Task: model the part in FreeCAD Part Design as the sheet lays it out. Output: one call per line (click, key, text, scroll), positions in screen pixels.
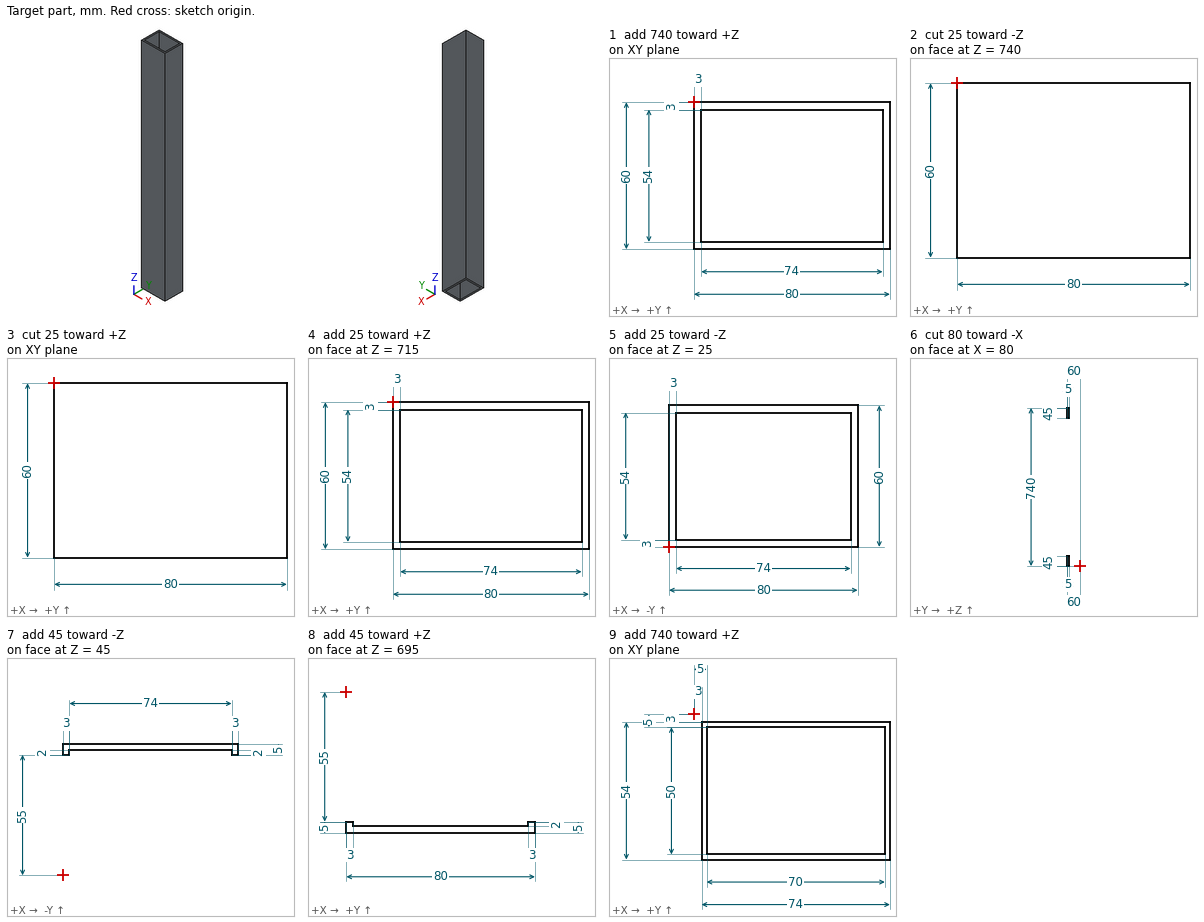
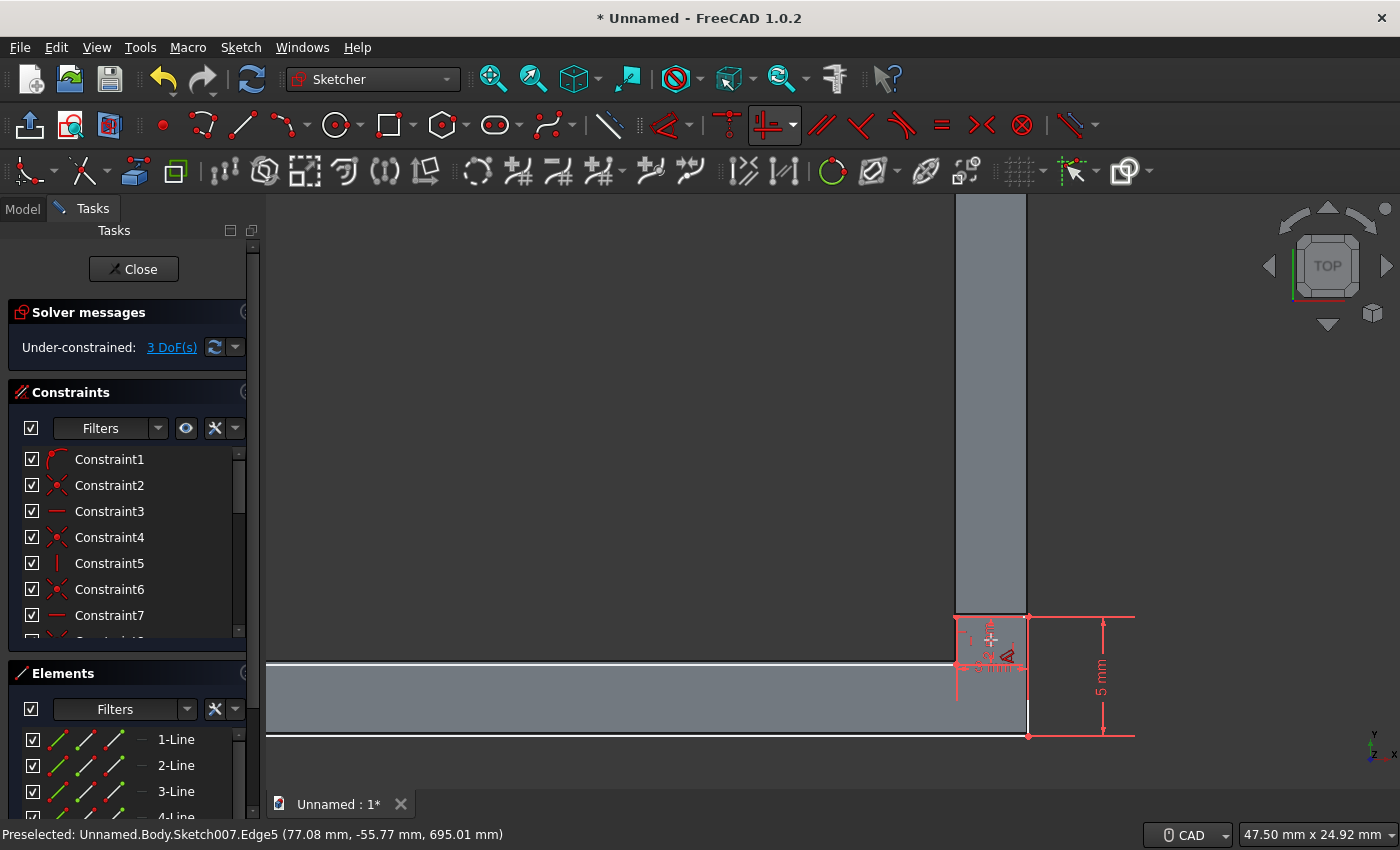
scroll(991, 647, down, 7)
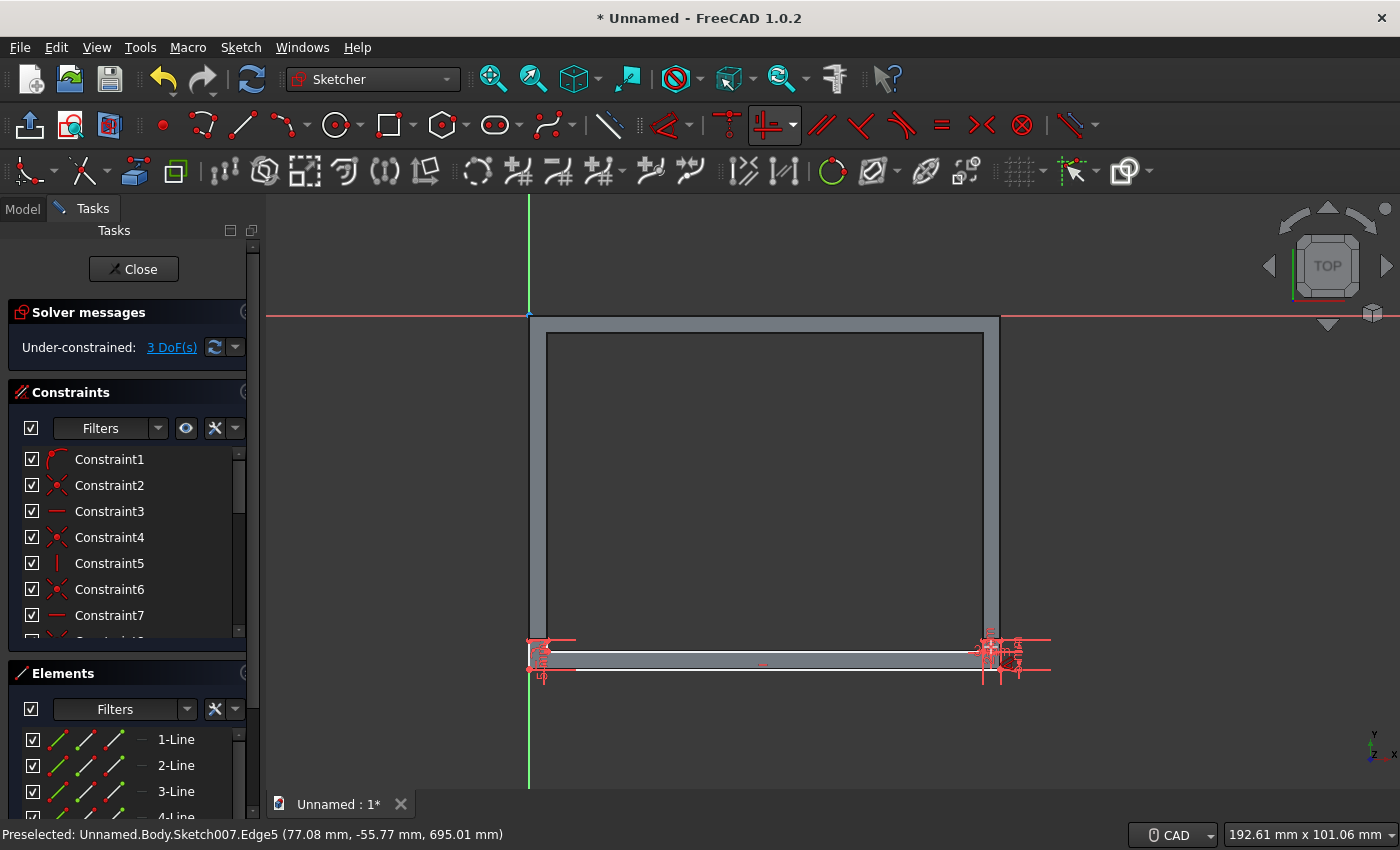
scroll(542, 640, up, 5)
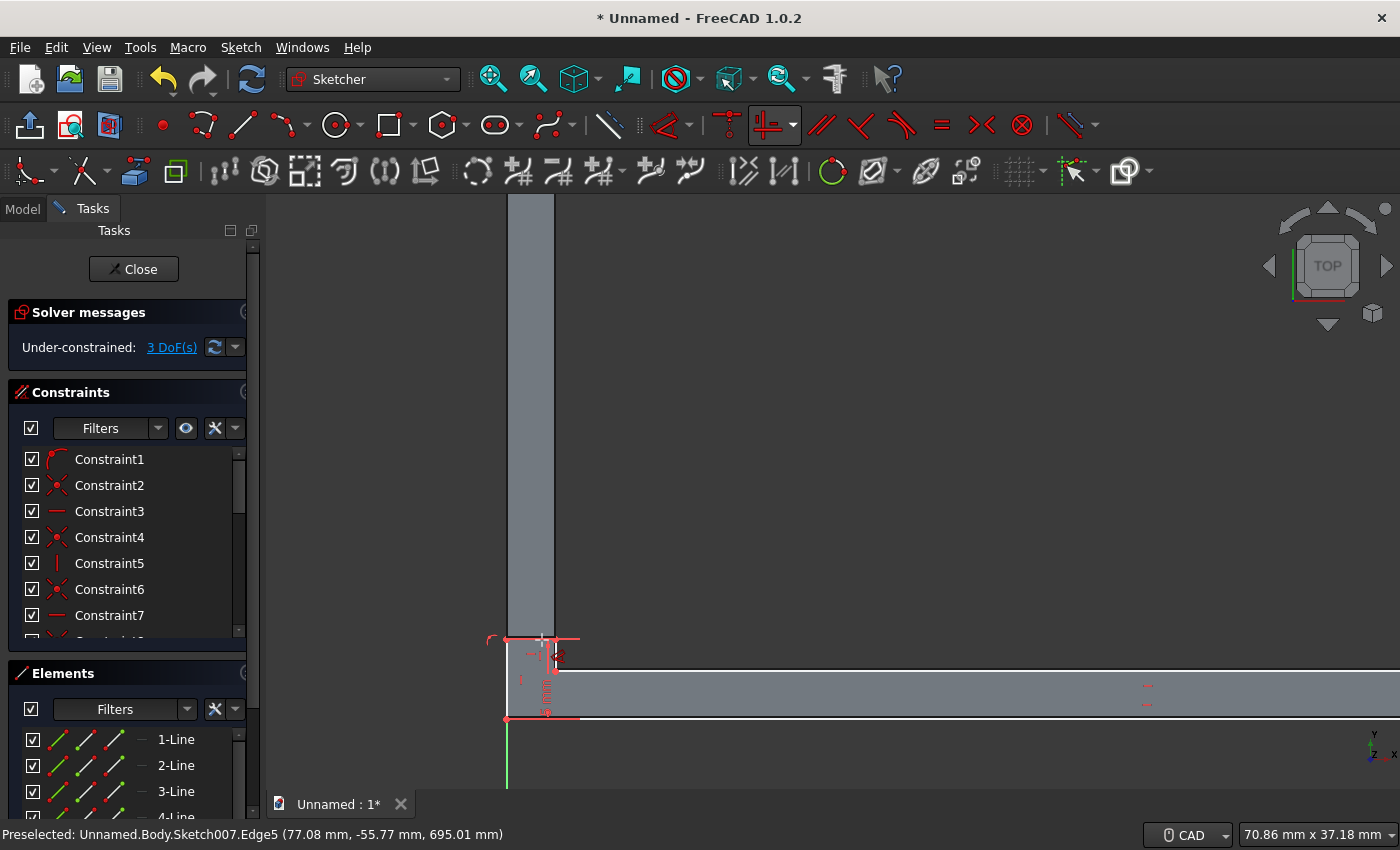
click(541, 639)
click(531, 673)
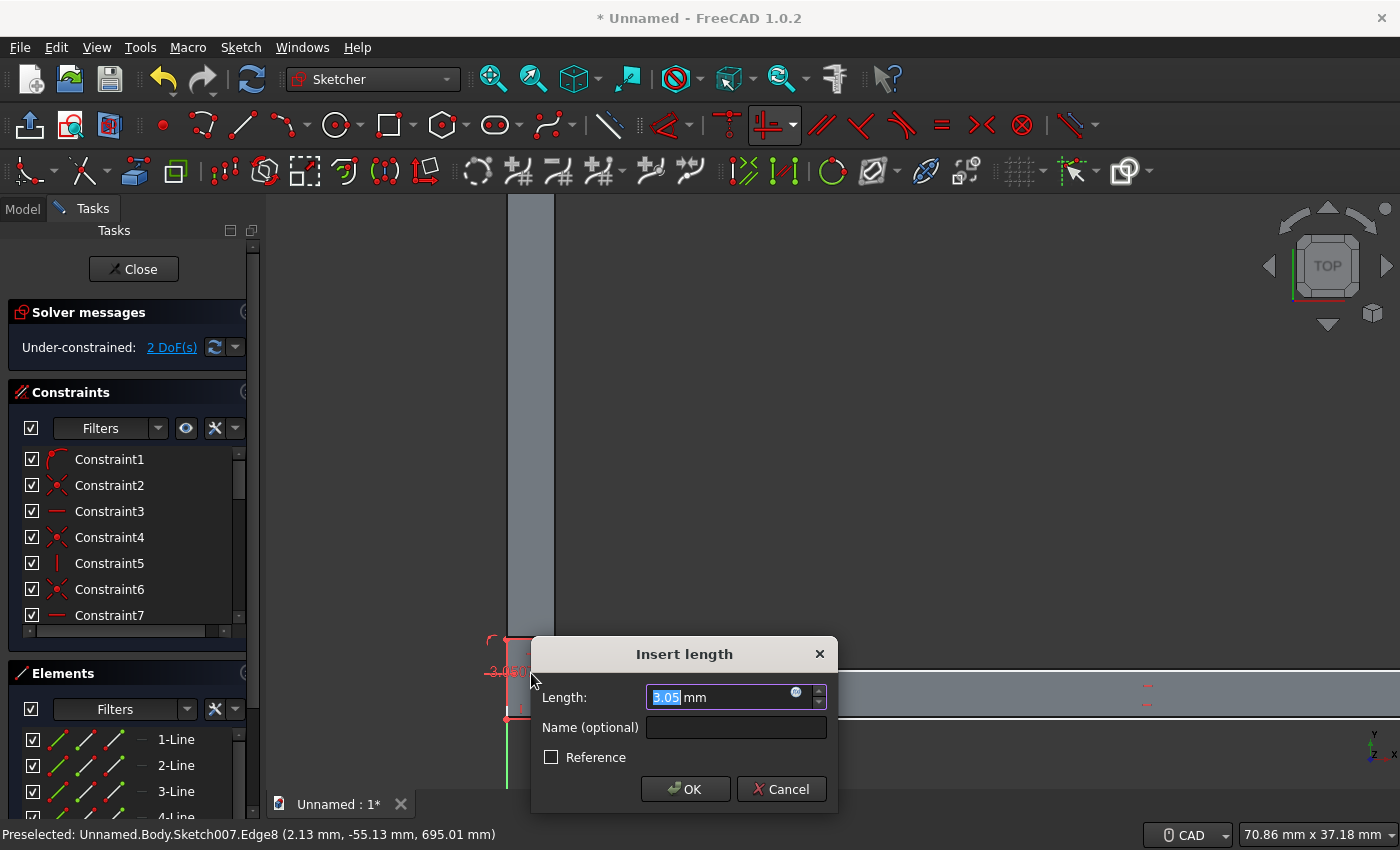
text(3)
key(Return)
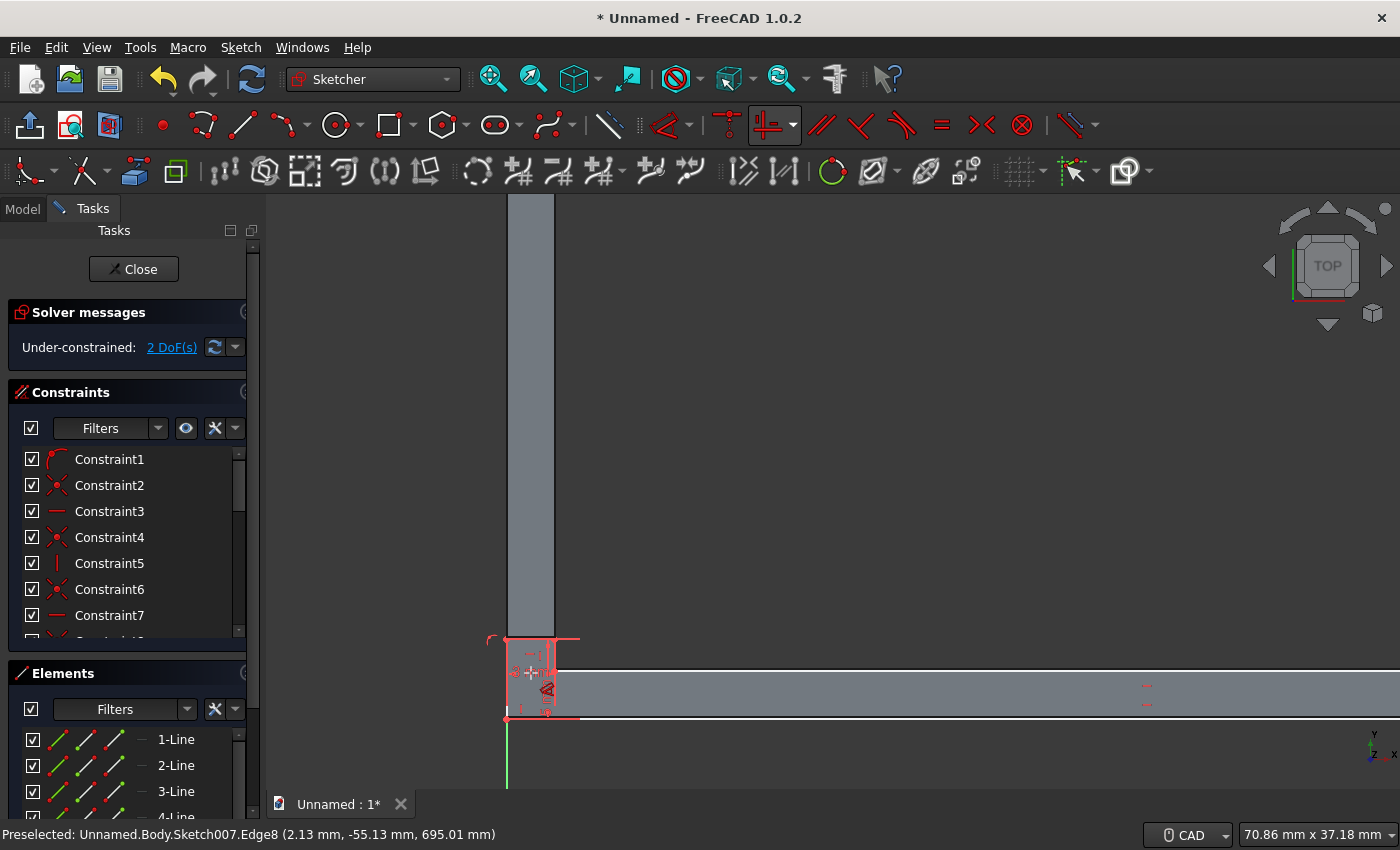
click(891, 719)
click(871, 753)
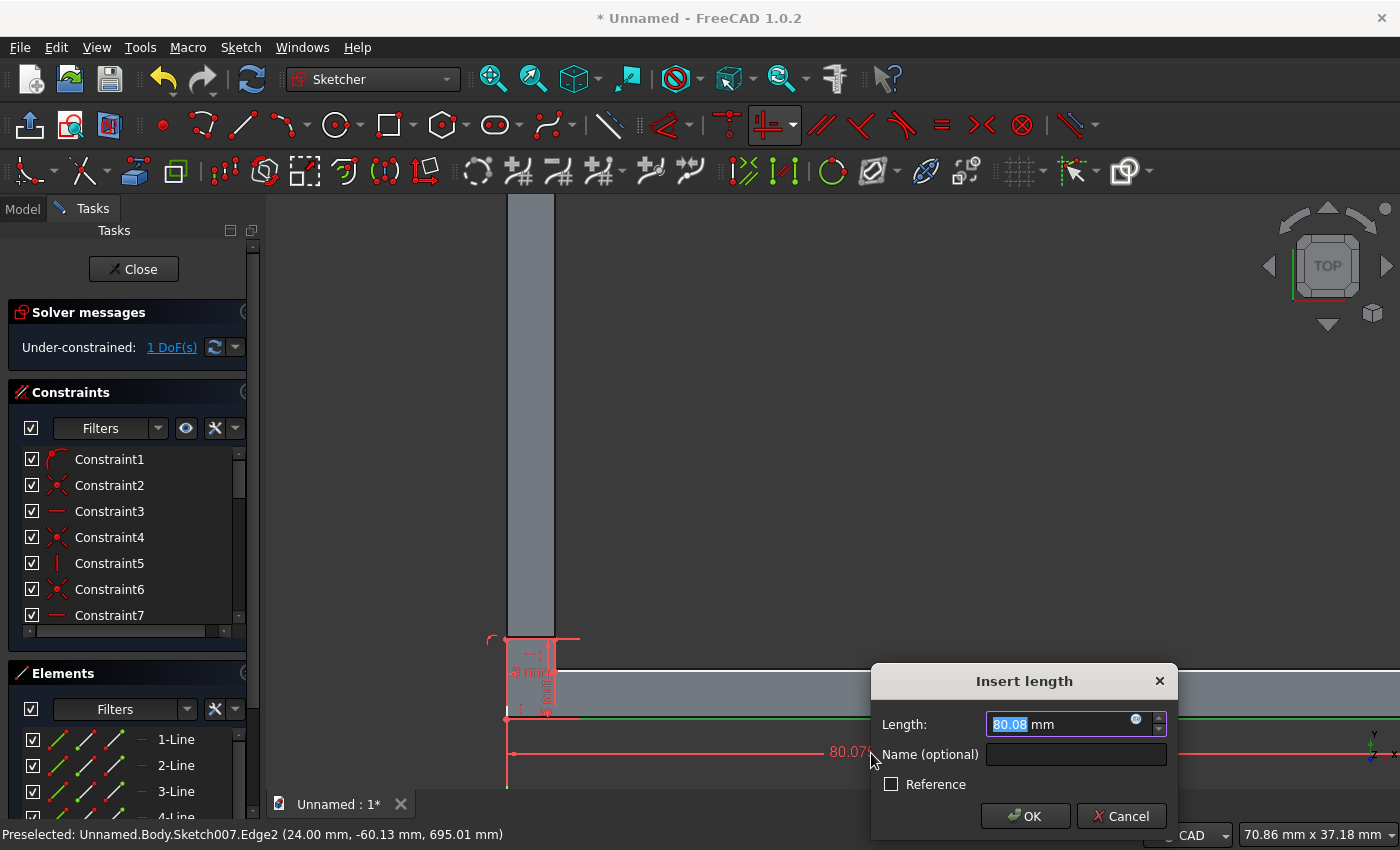
text(80)
key(Return)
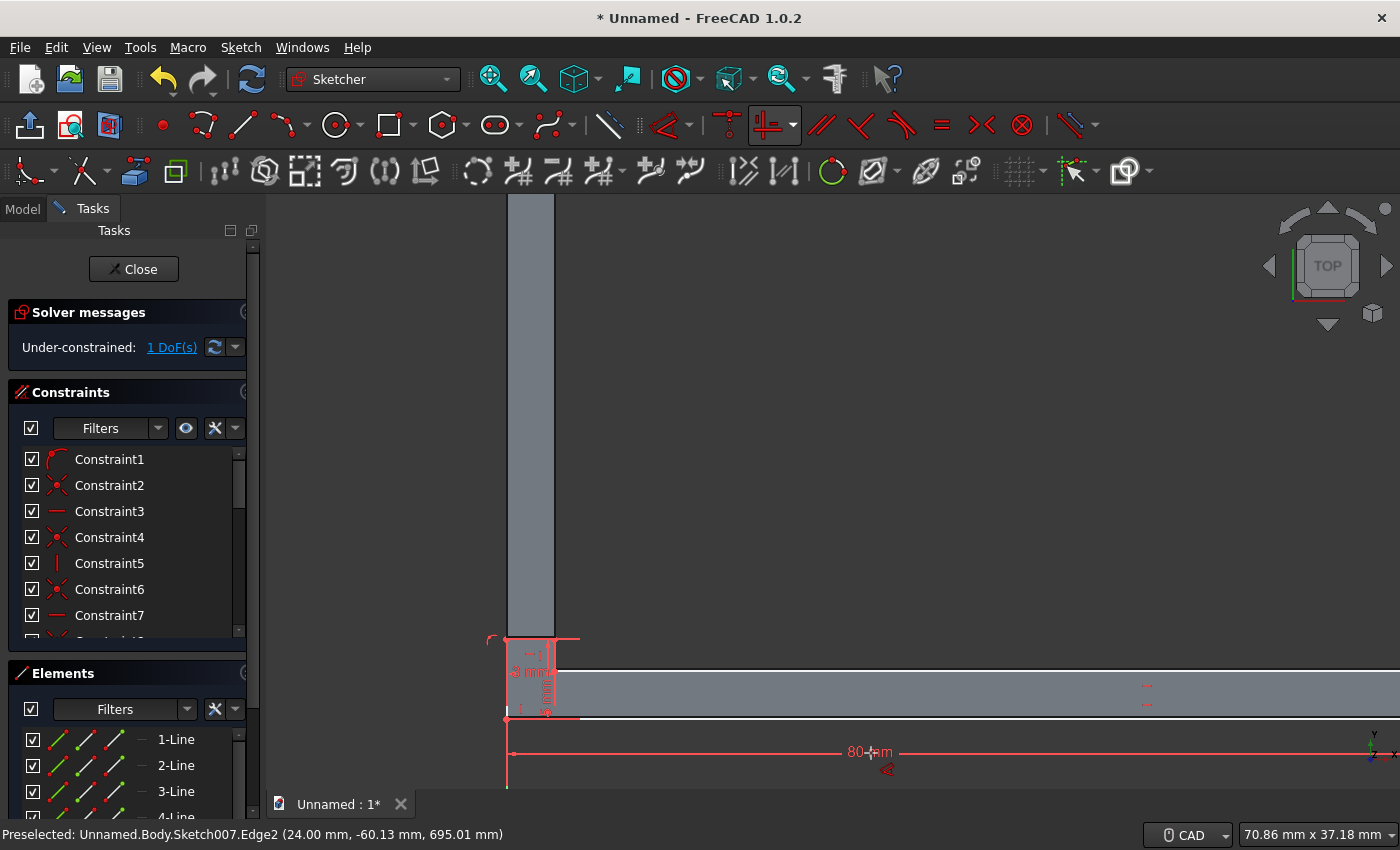
click(507, 639)
click(473, 431)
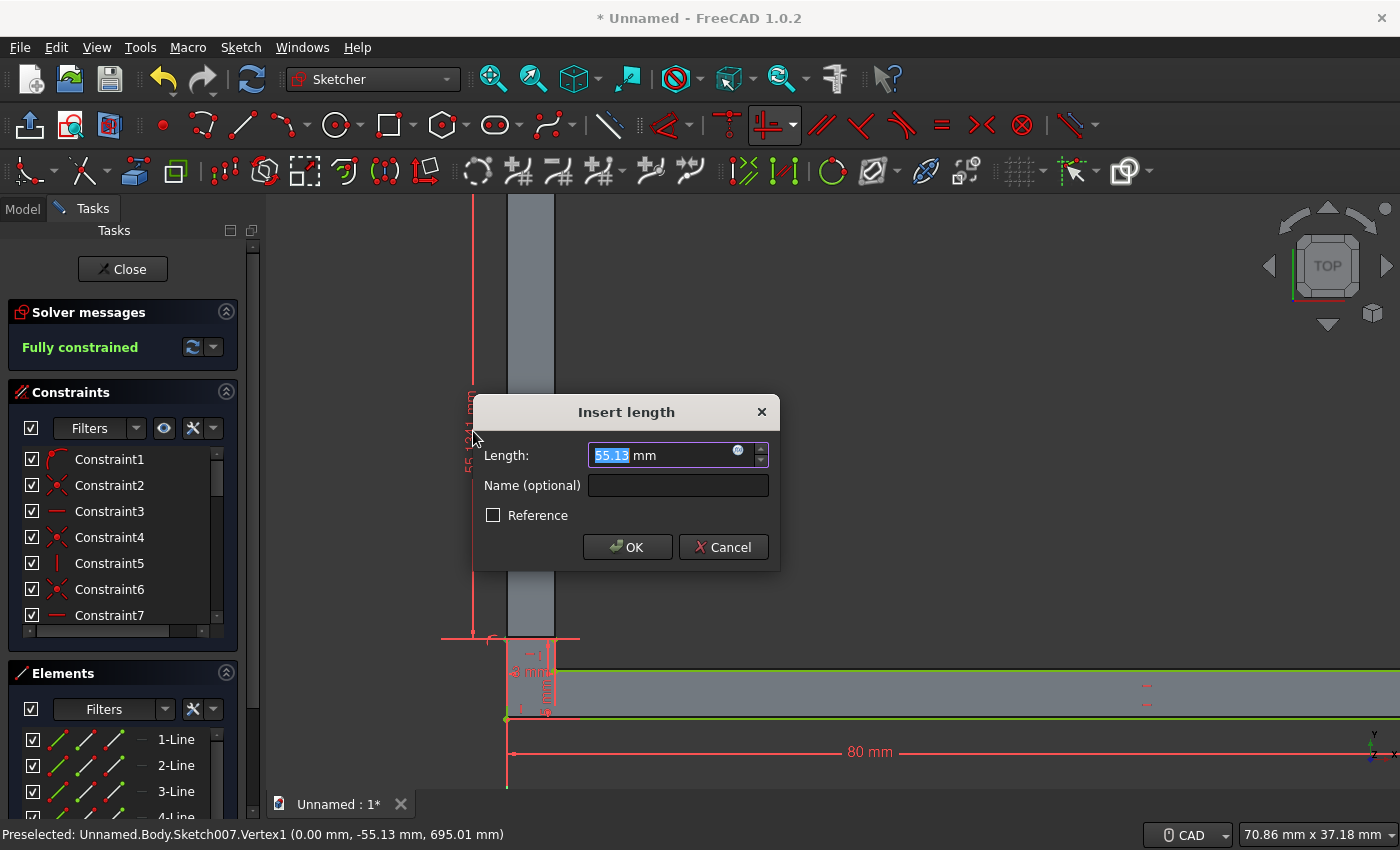
text(55)
key(Return)
key(Escape)